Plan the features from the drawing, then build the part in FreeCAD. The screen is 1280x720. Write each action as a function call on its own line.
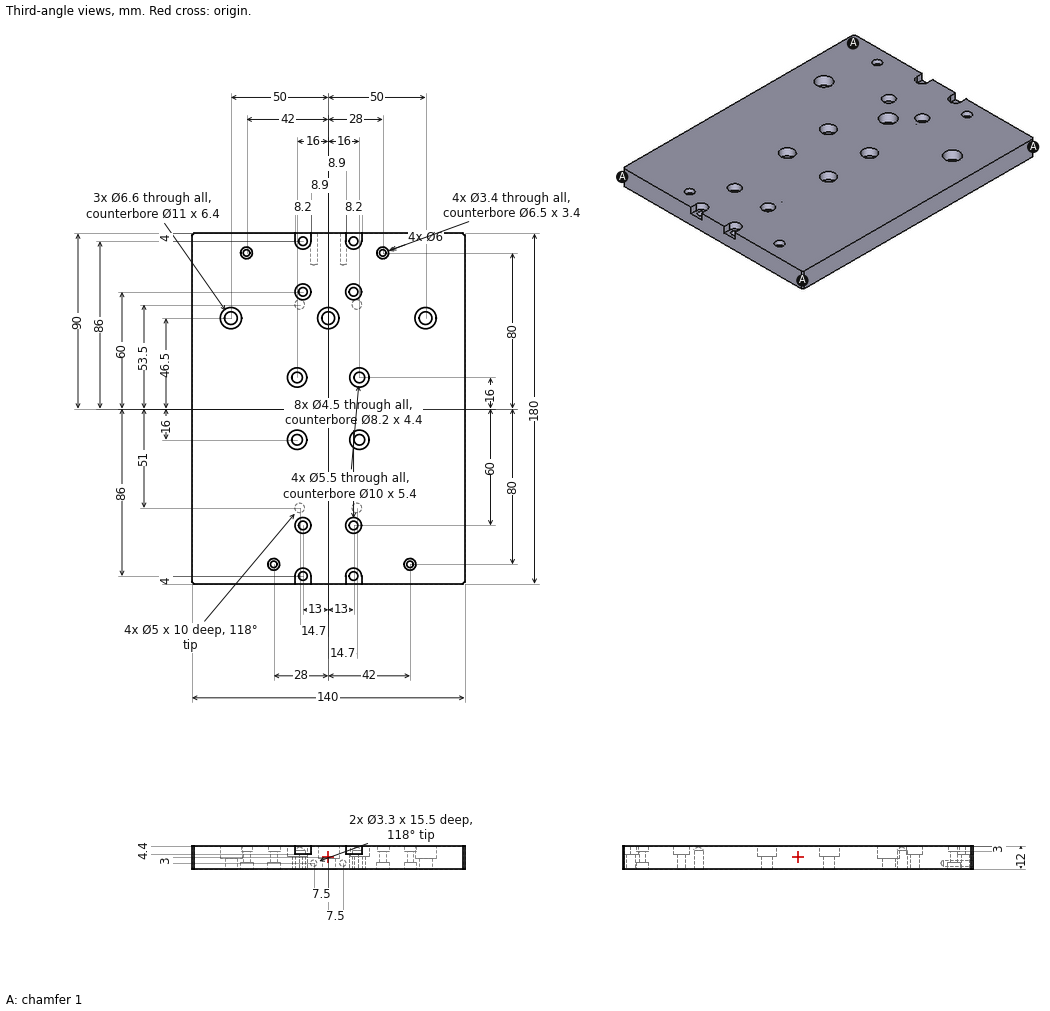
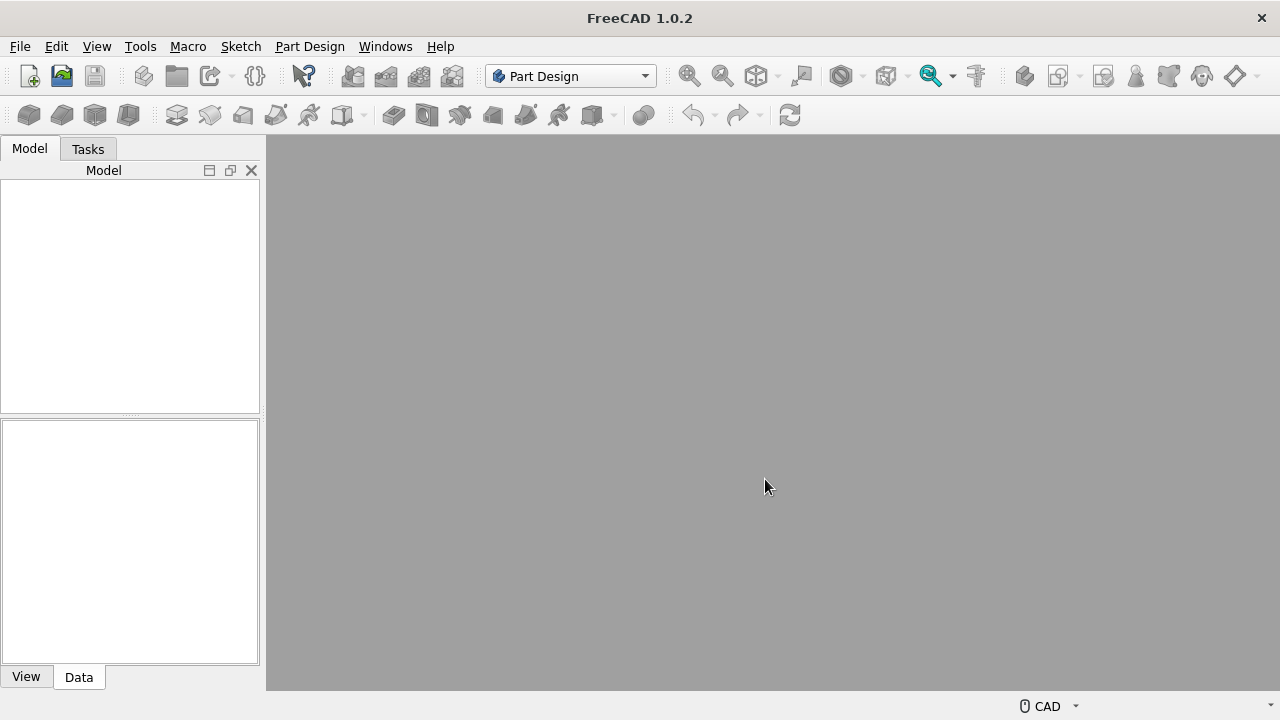
click(29, 76)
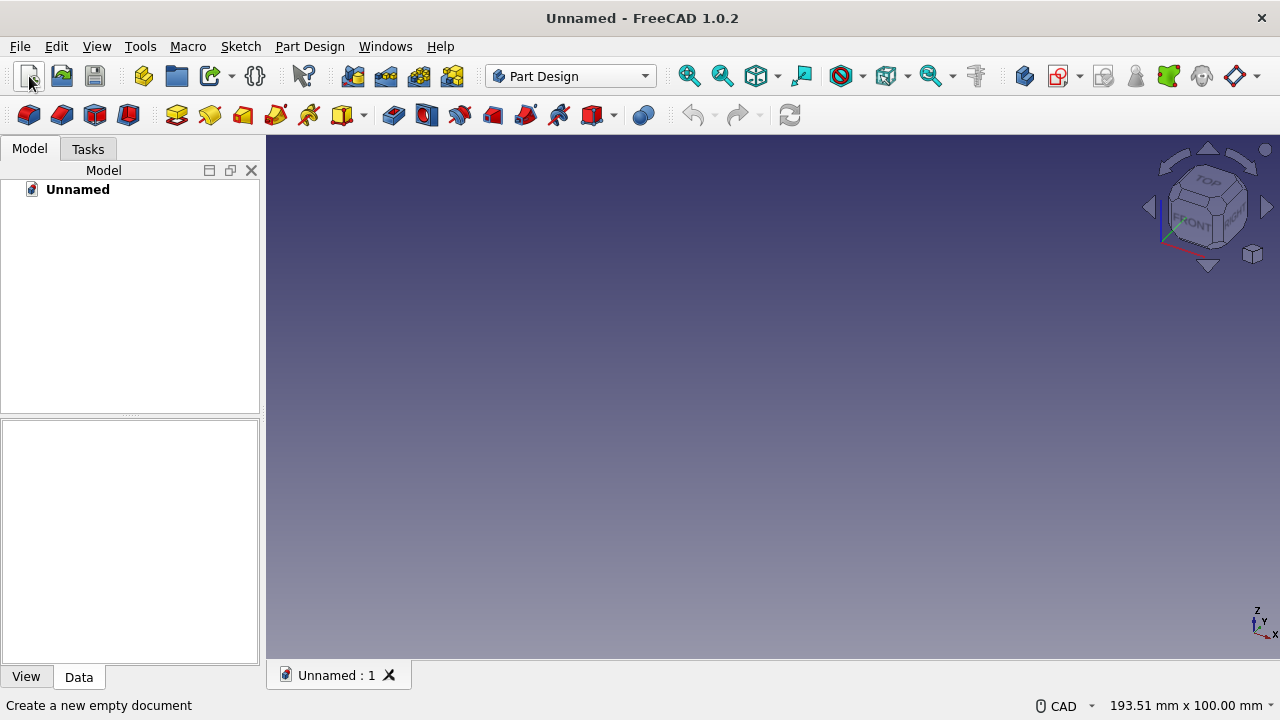
click(1058, 76)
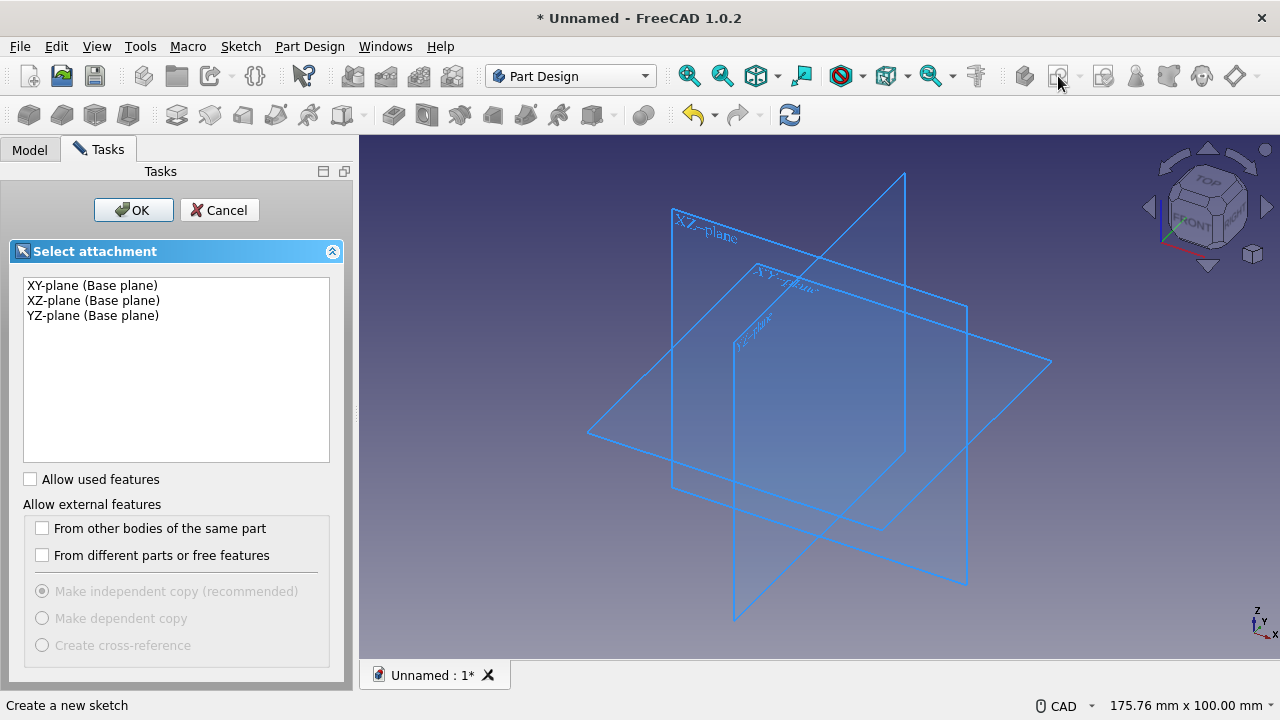
click(84, 286)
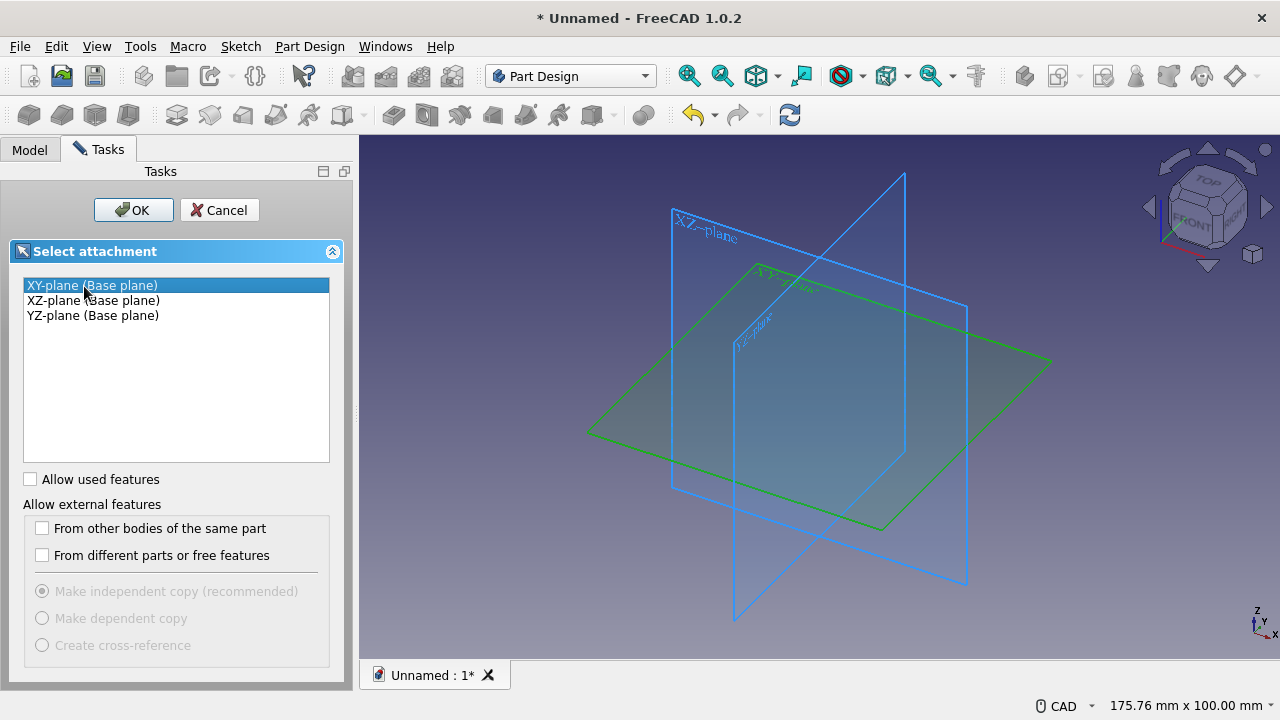
click(134, 210)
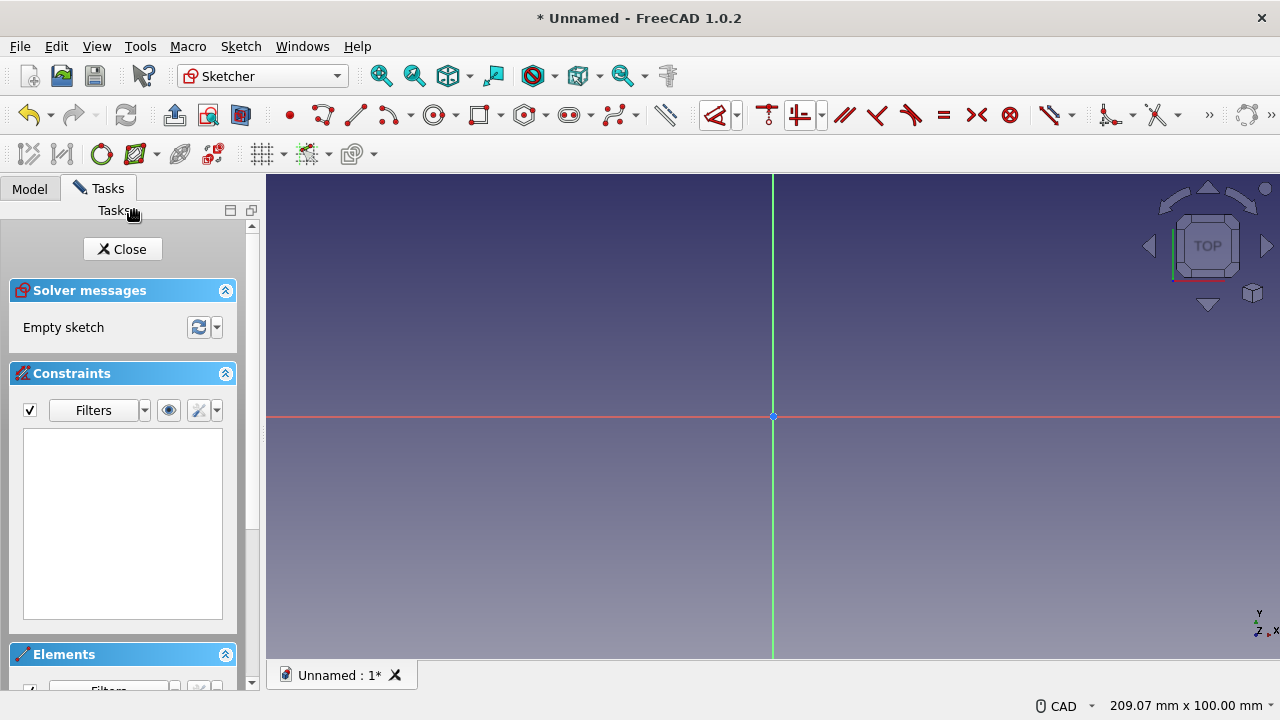
scroll(665, 417, down, 5)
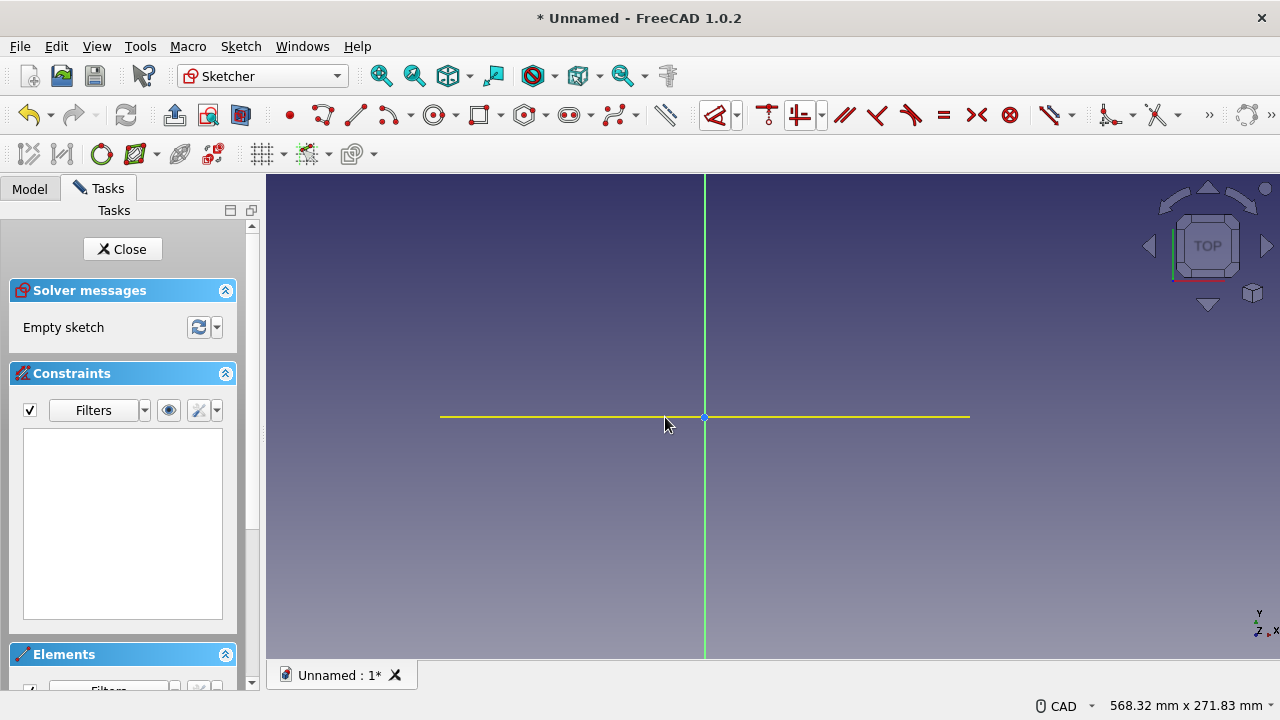
click(500, 116)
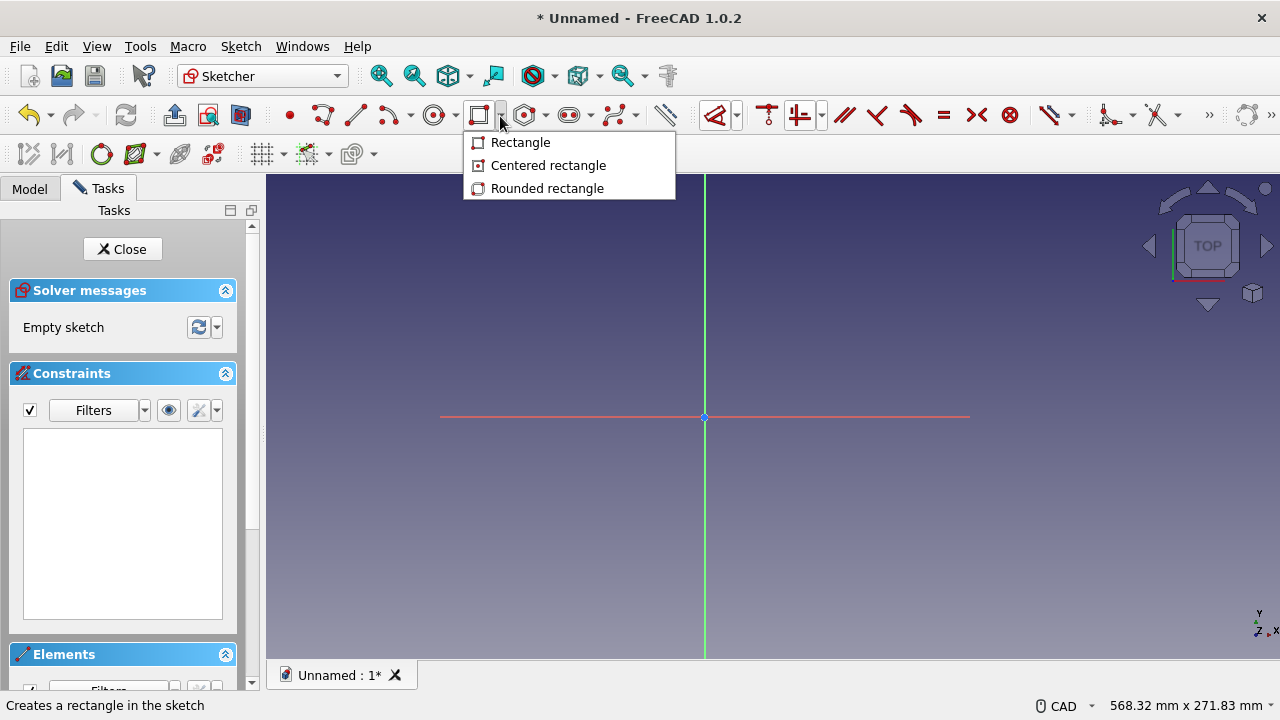
click(570, 166)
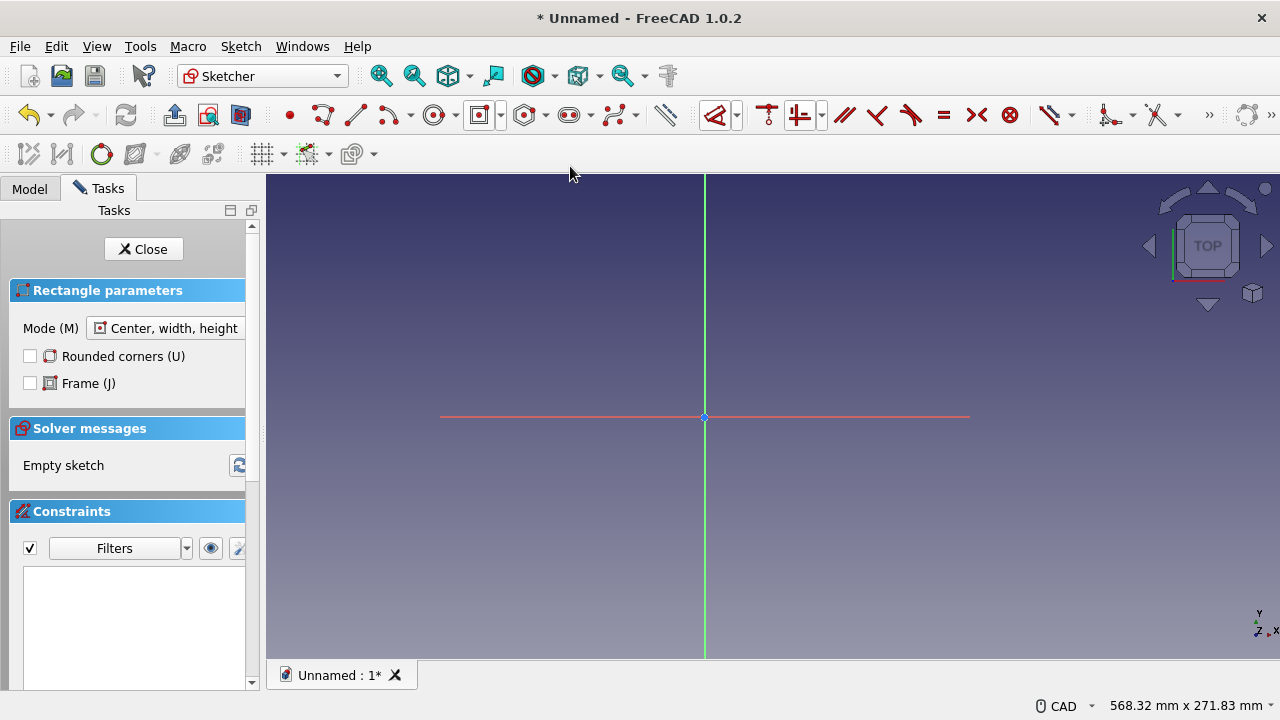
click(705, 417)
click(830, 257)
key(Escape)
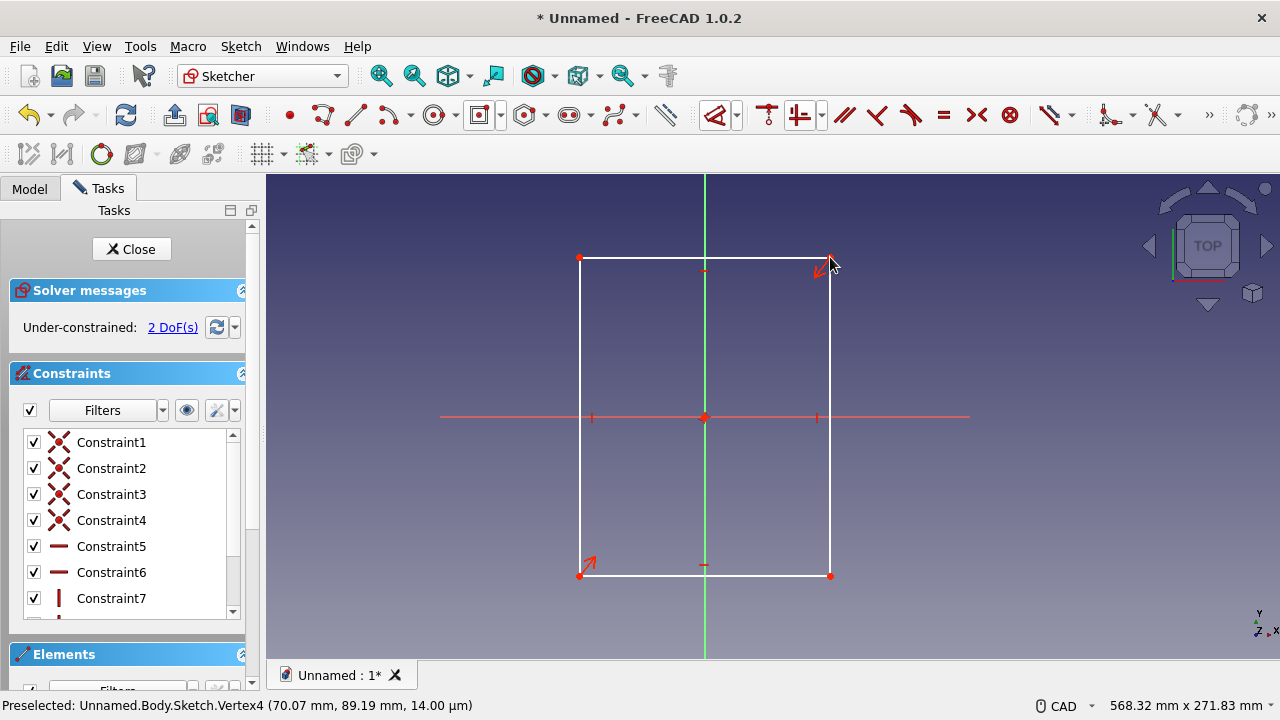
click(714, 116)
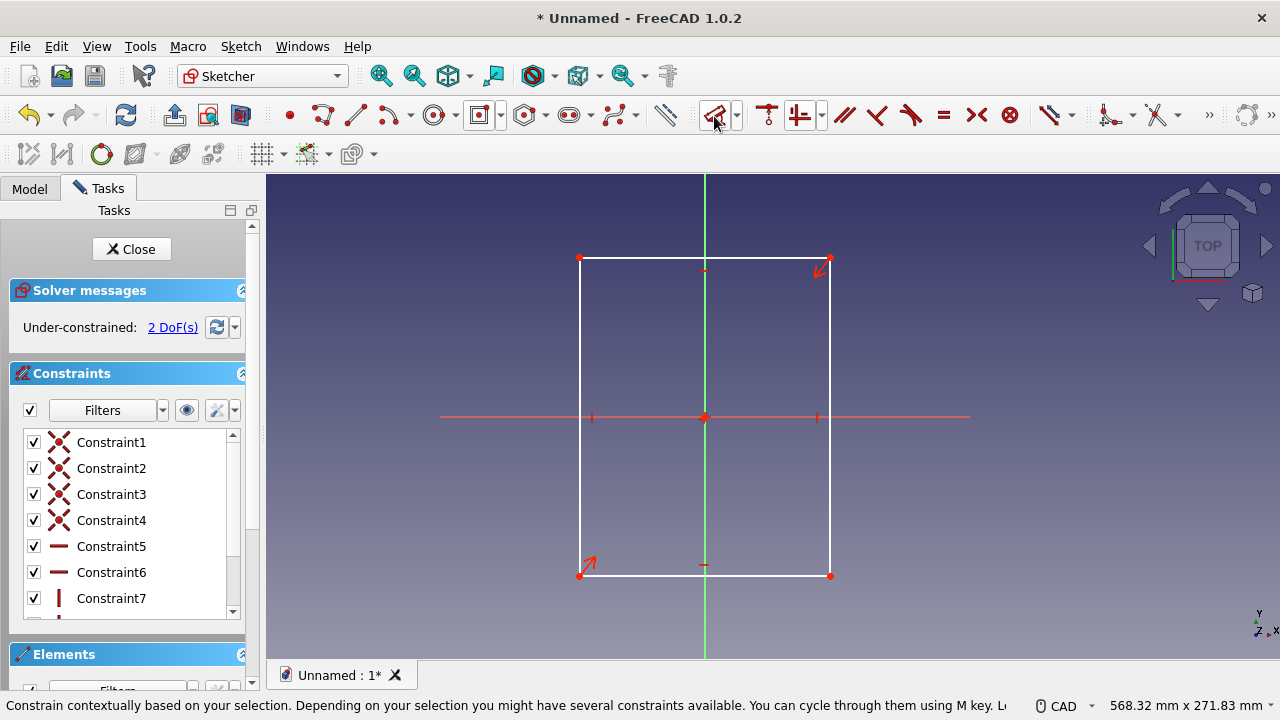
click(655, 576)
click(647, 610)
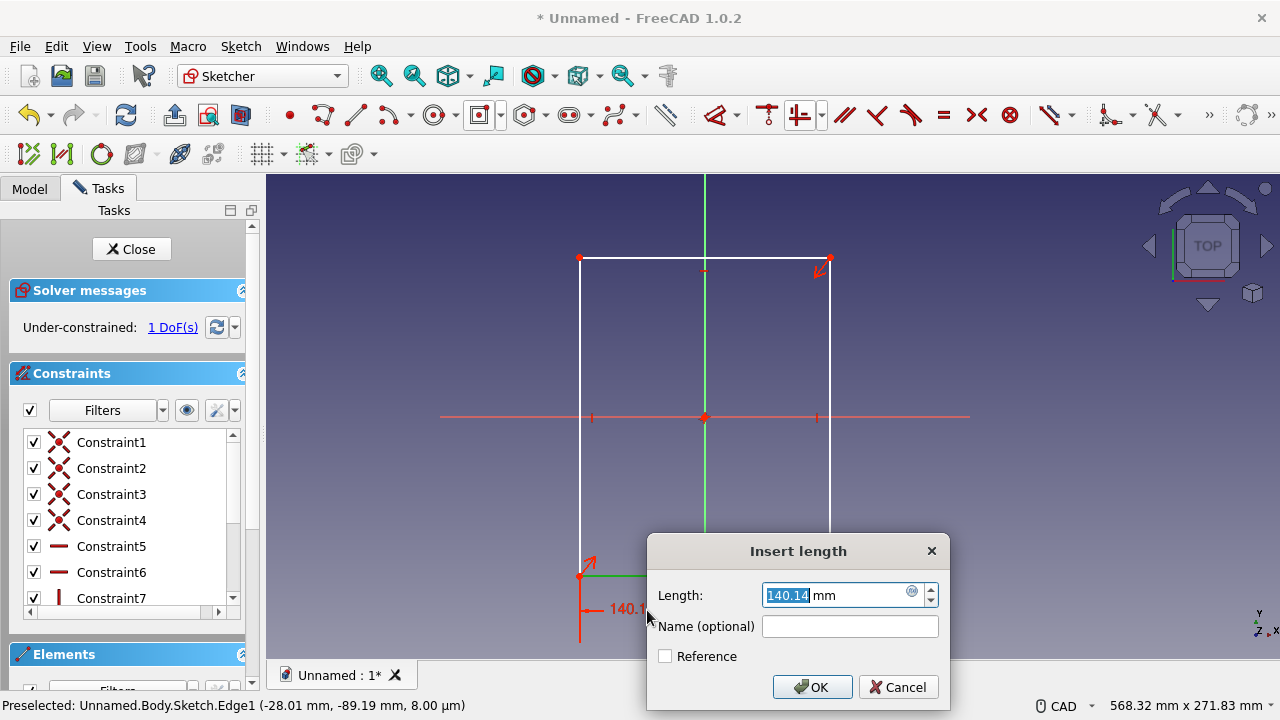
text(140)
key(Return)